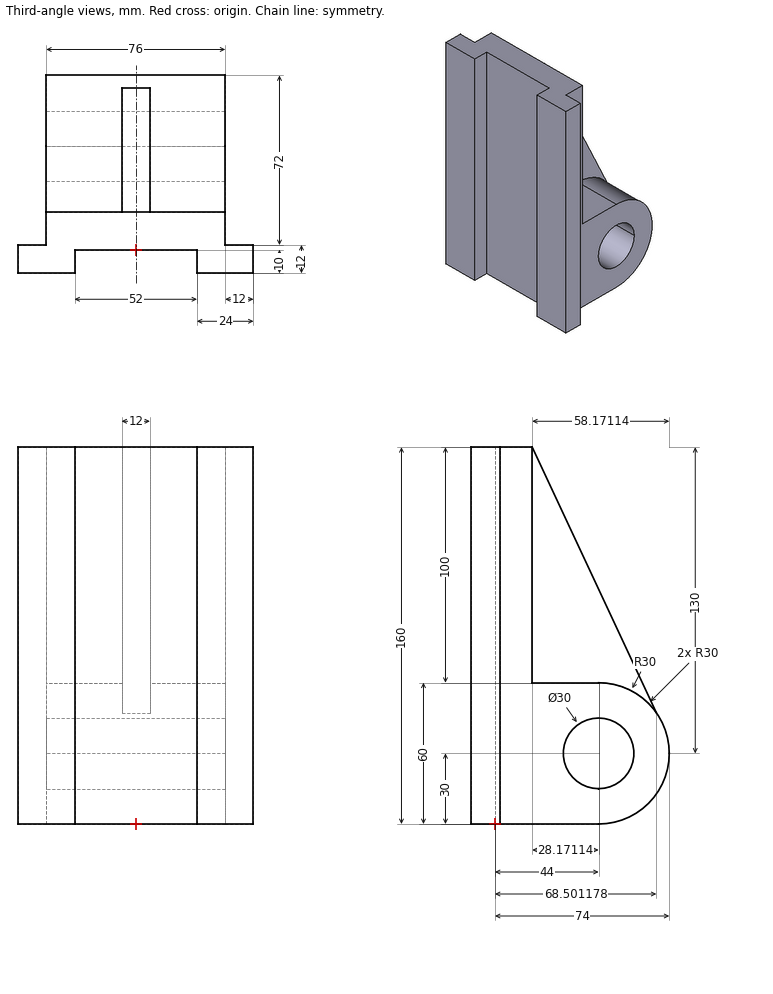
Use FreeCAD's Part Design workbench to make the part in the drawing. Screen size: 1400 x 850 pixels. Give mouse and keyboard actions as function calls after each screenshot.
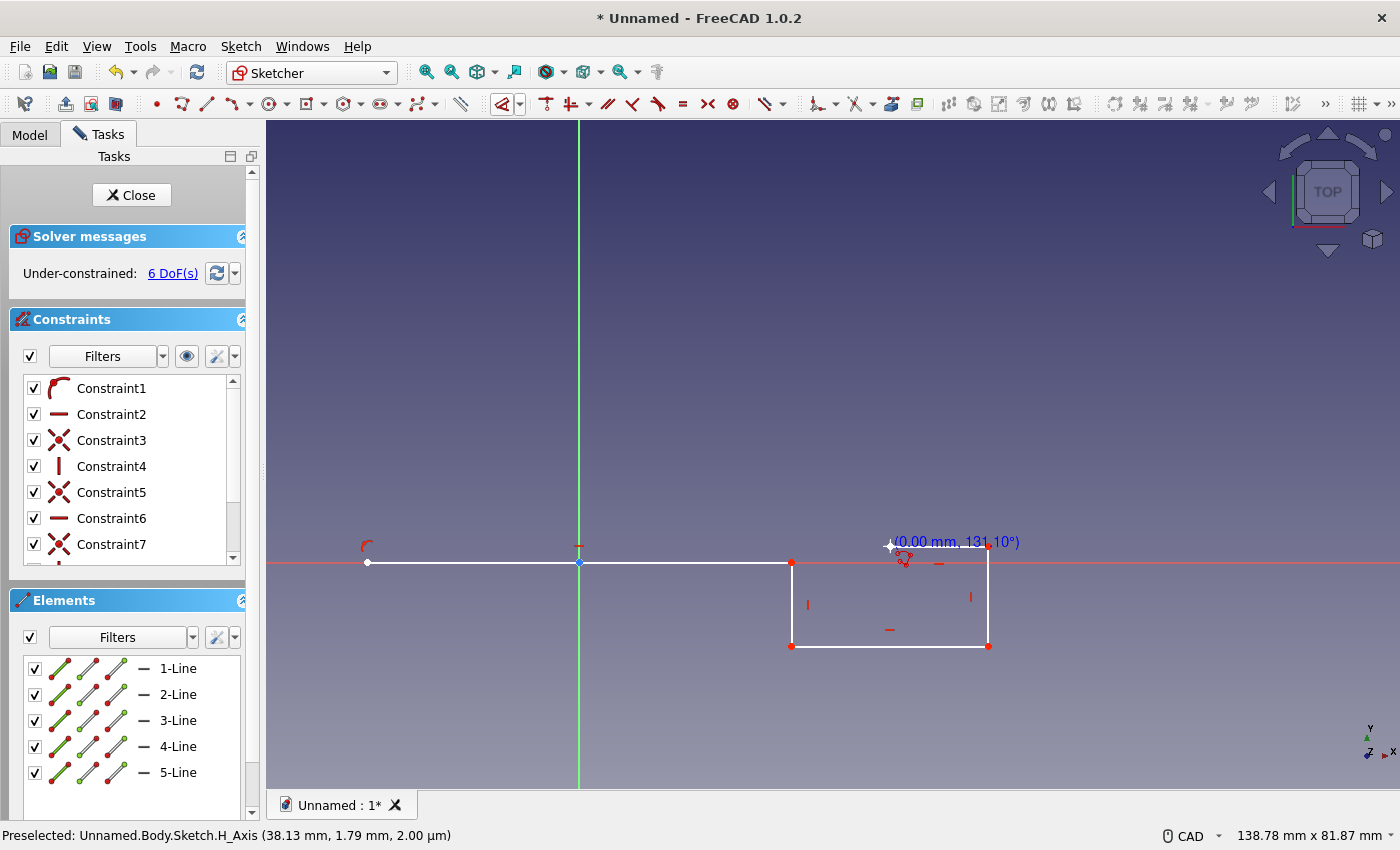
scroll(1141, 761, down, 2)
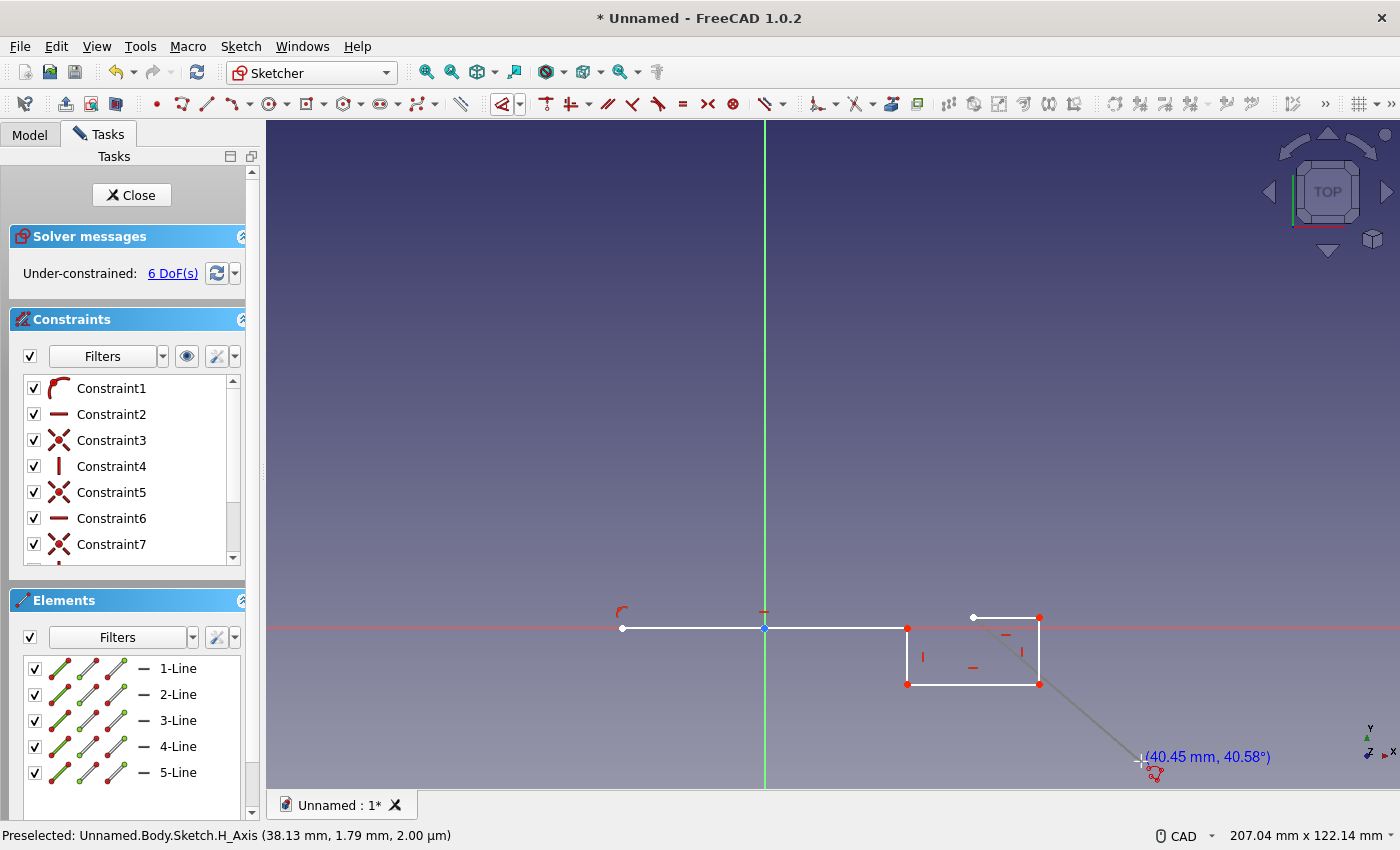
click(973, 223)
click(557, 223)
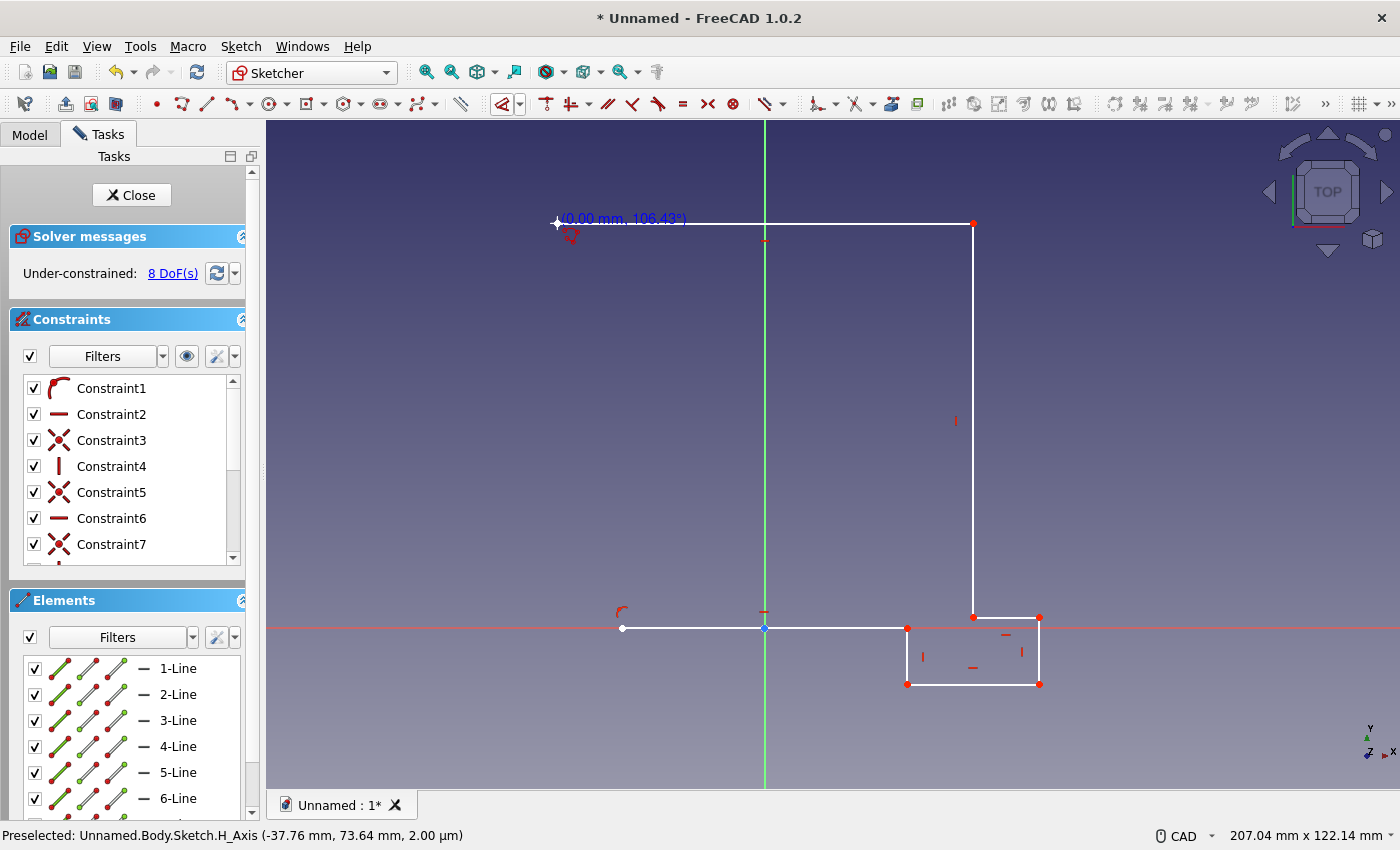
scroll(557, 617, up, 2)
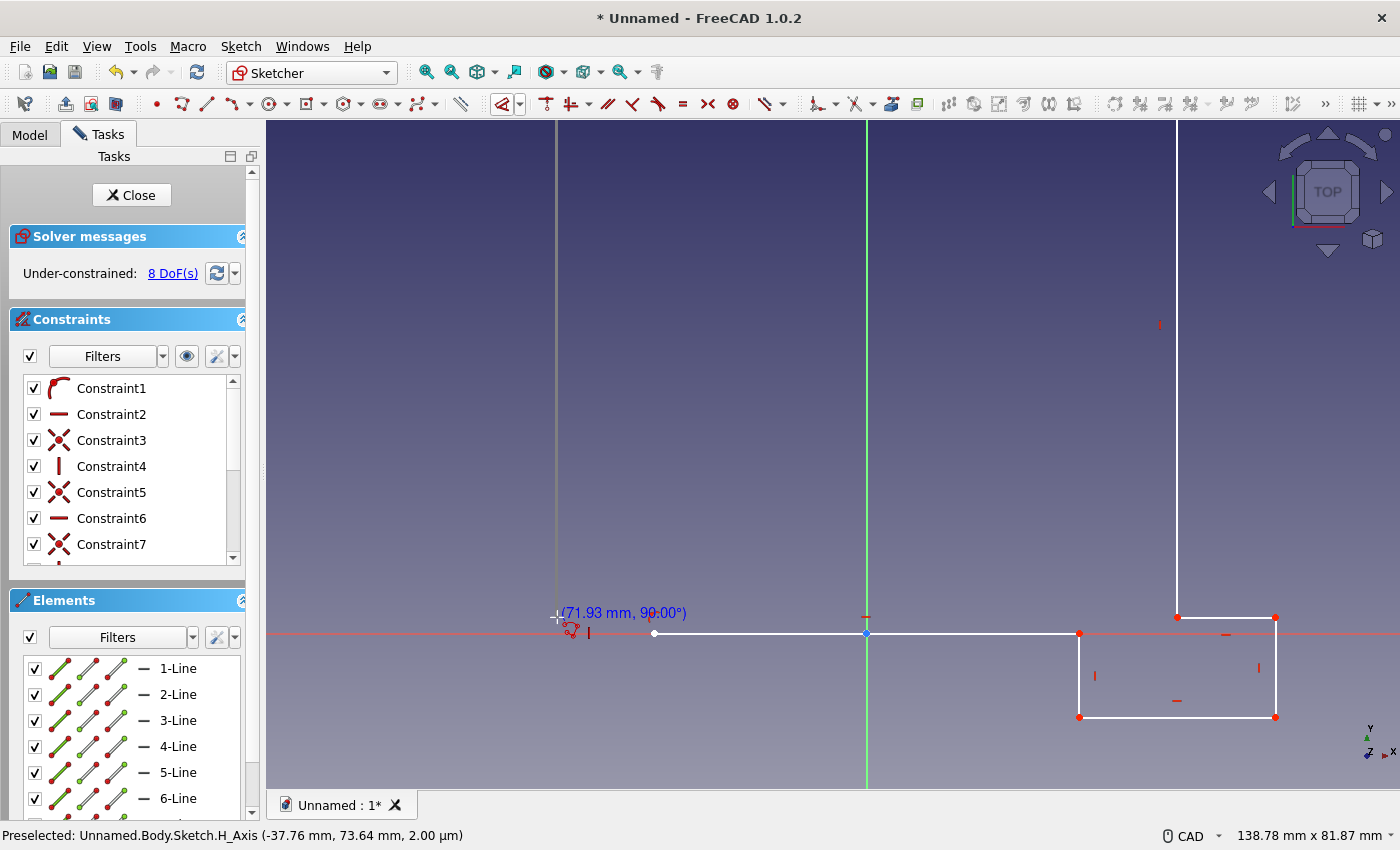
click(557, 617)
click(458, 617)
click(458, 715)
click(654, 715)
click(655, 634)
key(Escape)
key(Escape)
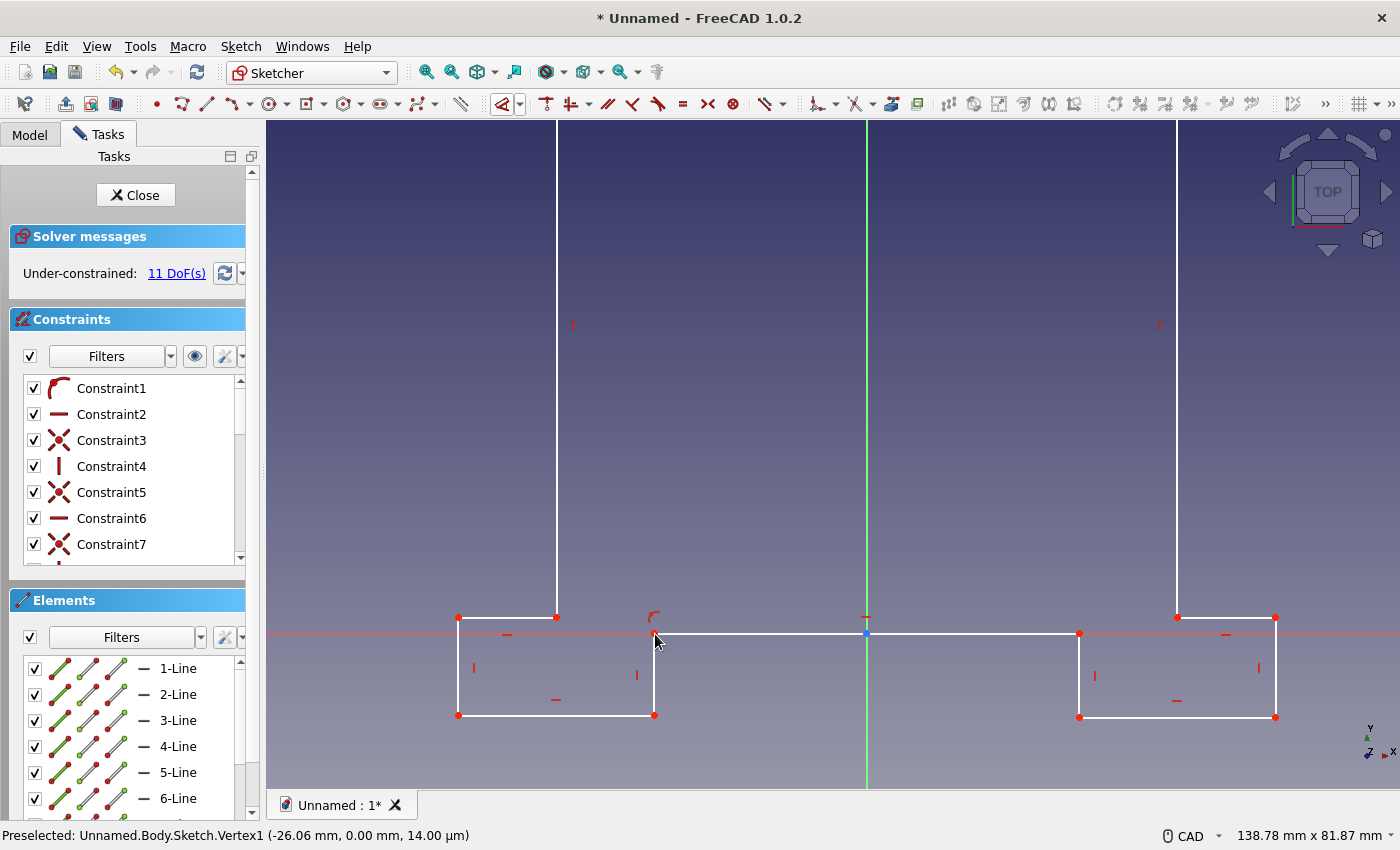
click(1177, 618)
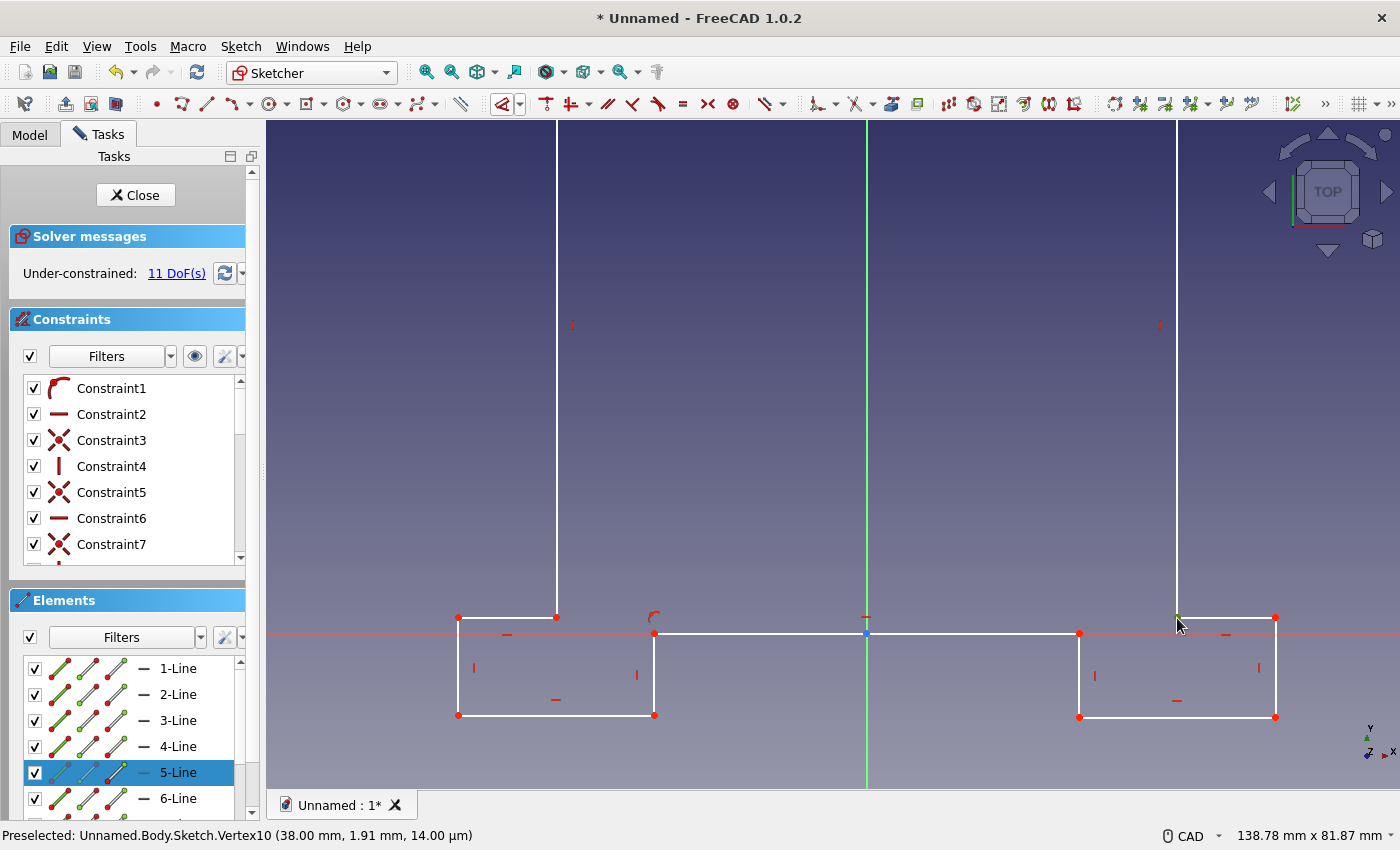
click(557, 618)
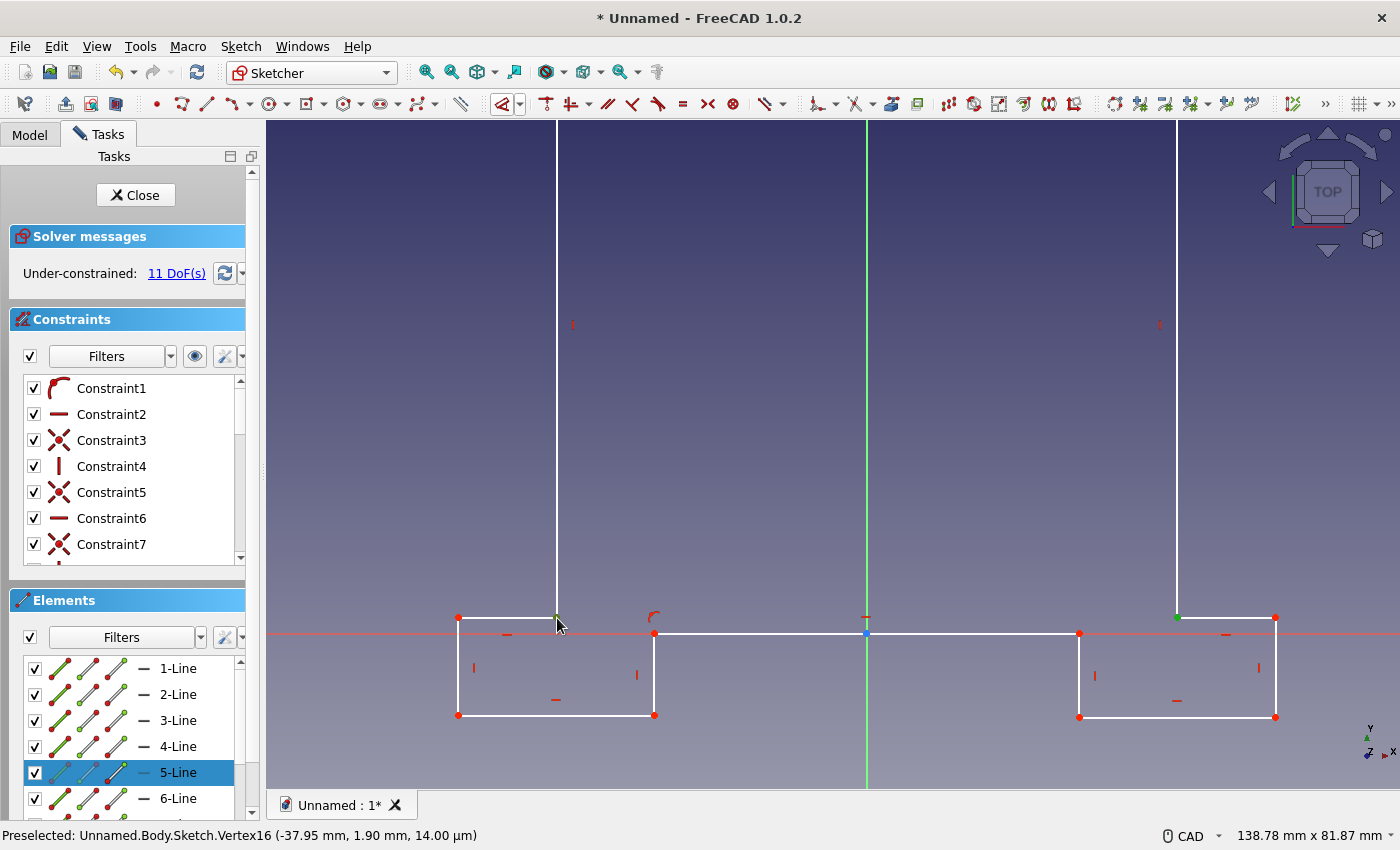
click(867, 717)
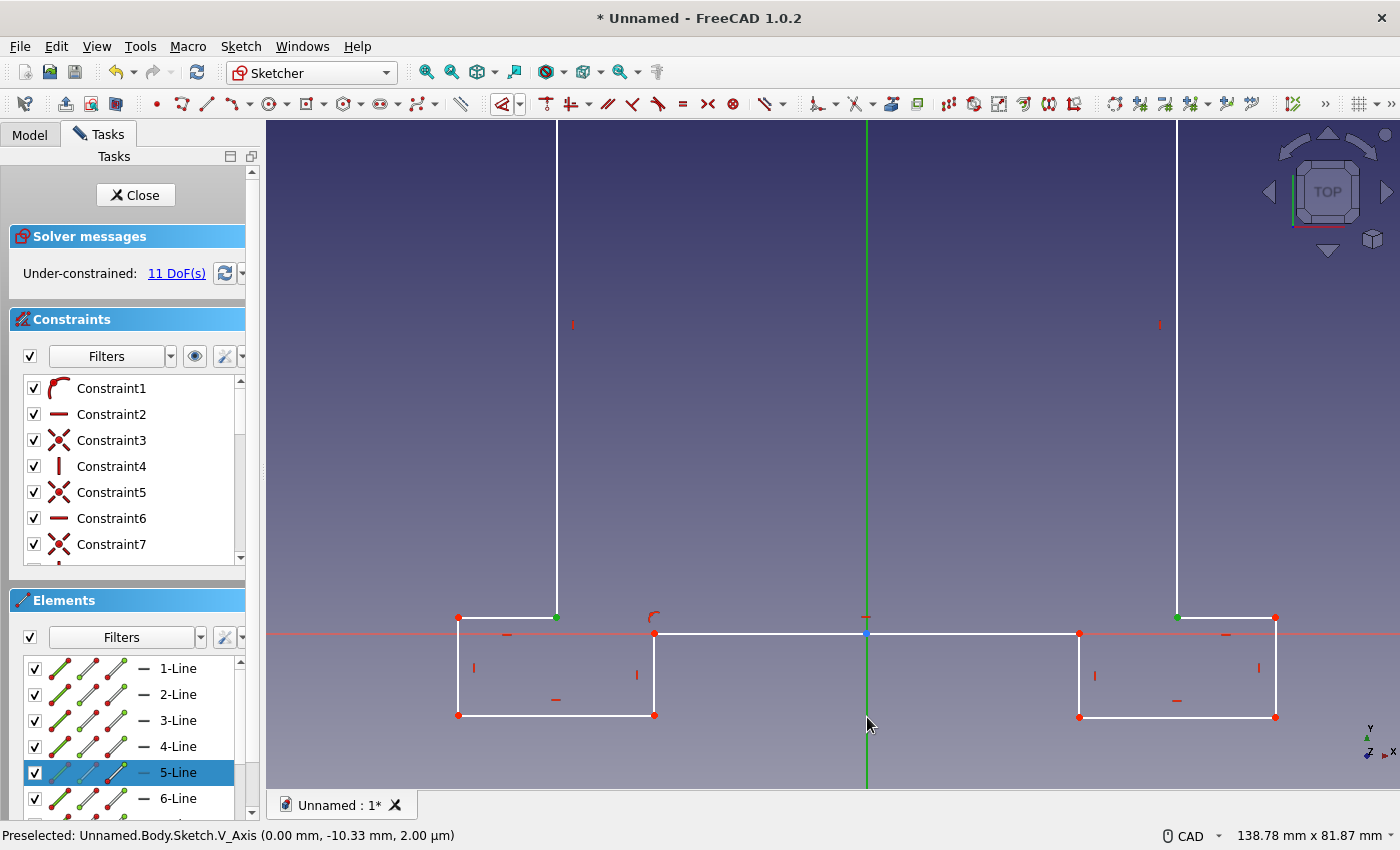
click(708, 104)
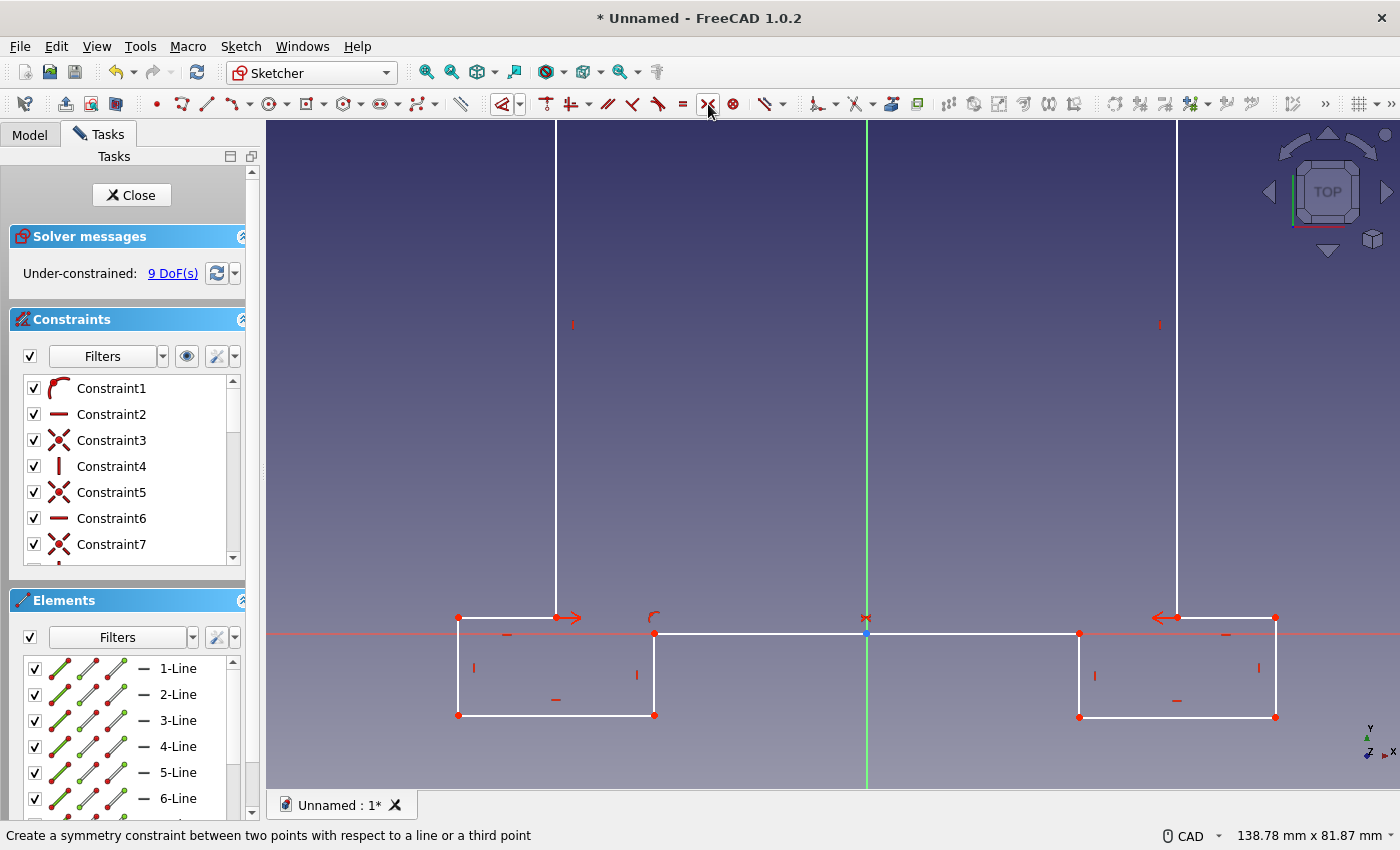
scroll(556, 622, down, 2)